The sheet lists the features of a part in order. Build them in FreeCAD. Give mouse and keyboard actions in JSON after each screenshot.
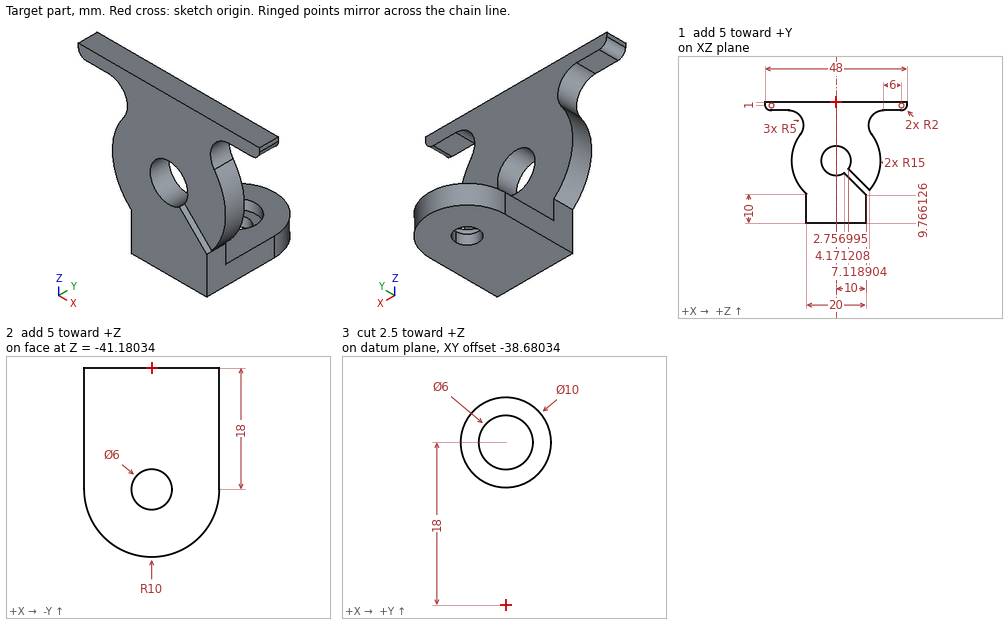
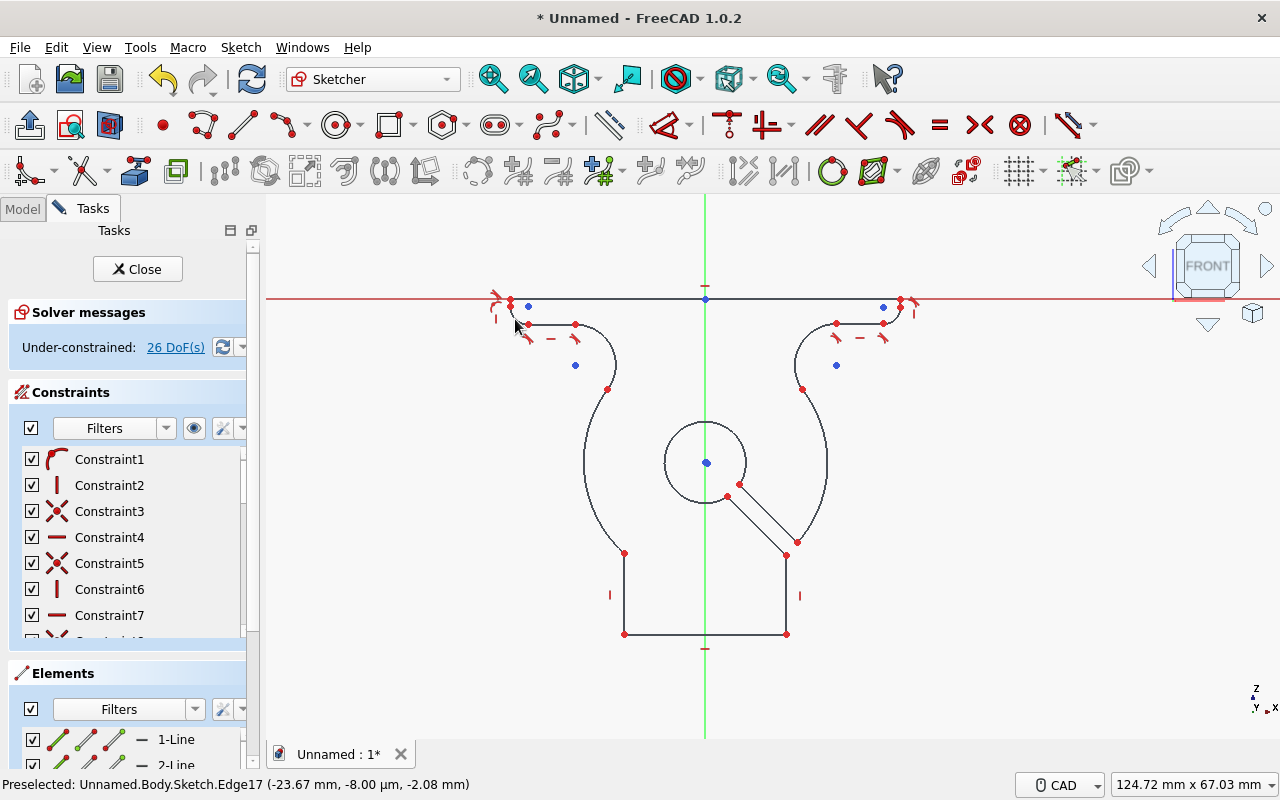
{"action": "left_click", "coordinate": [811, 333]}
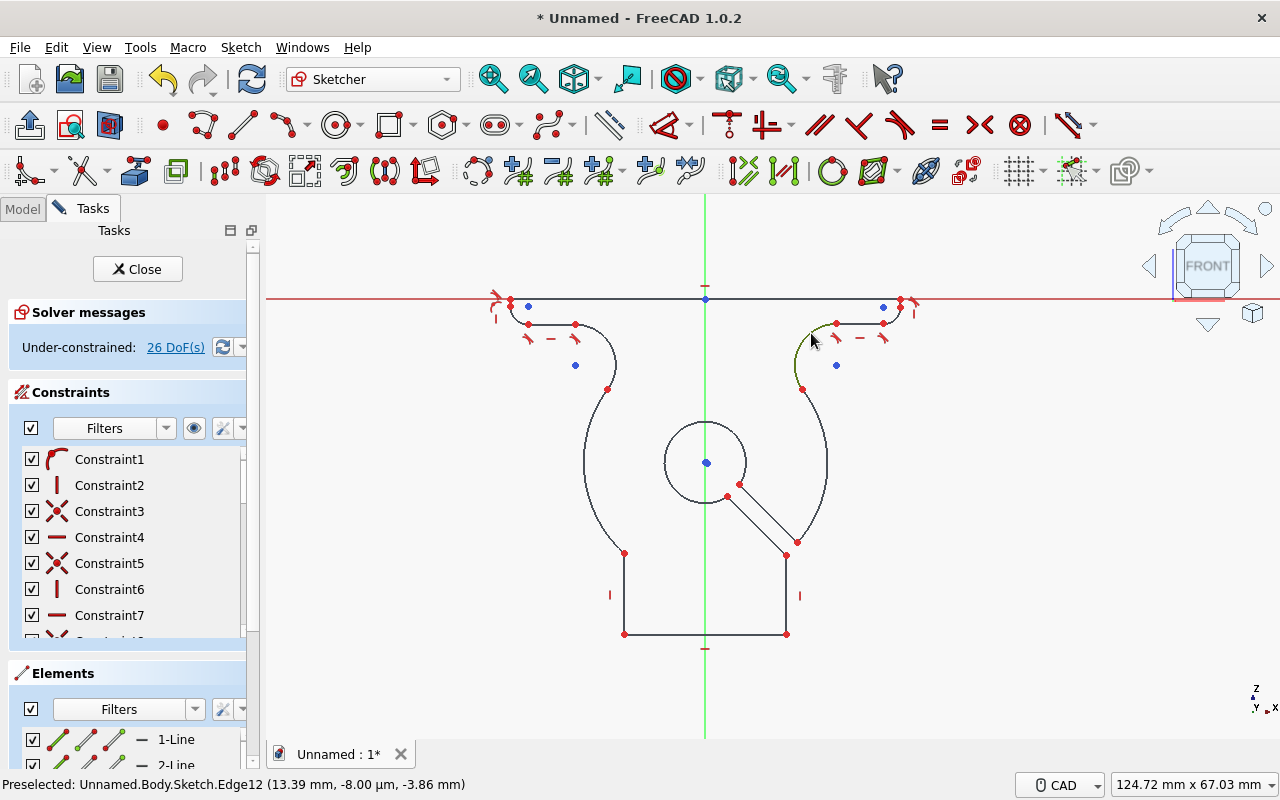
{"action": "left_click", "coordinate": [822, 500]}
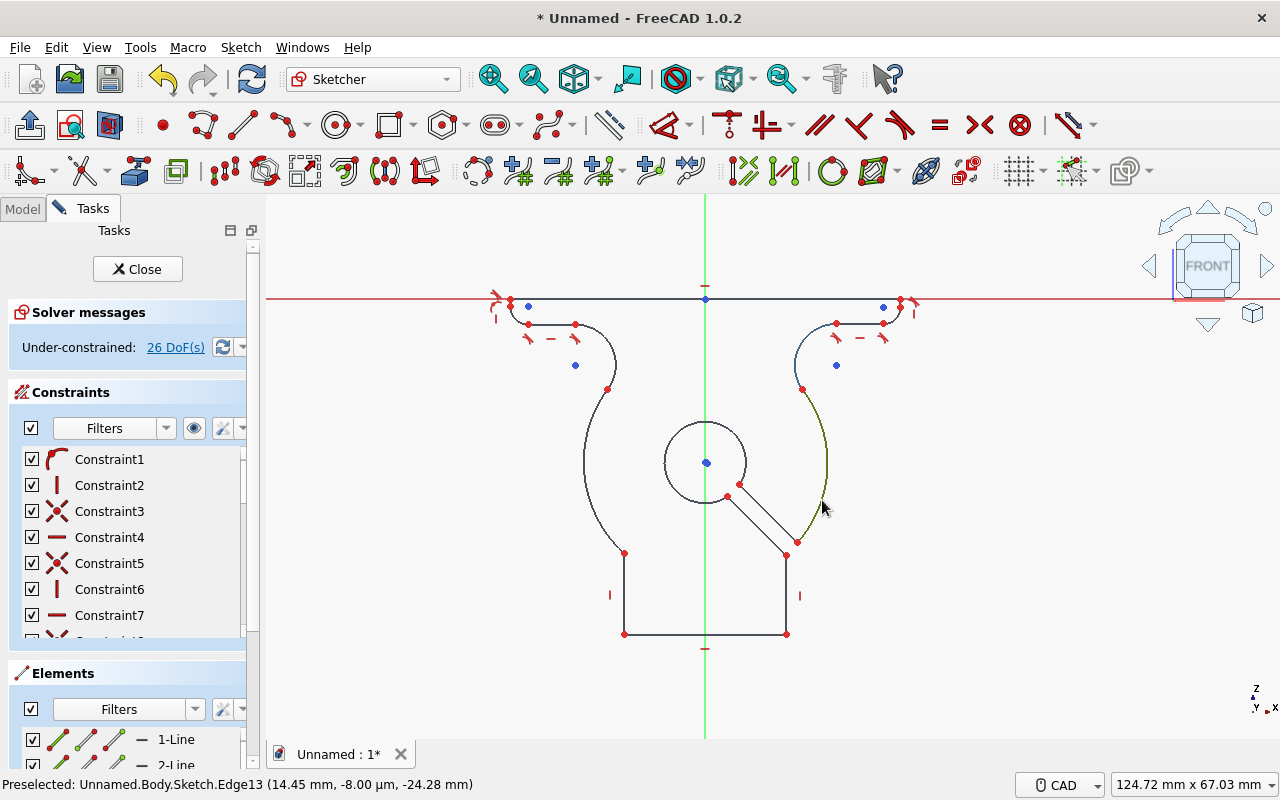
{"action": "left_click", "coordinate": [900, 126]}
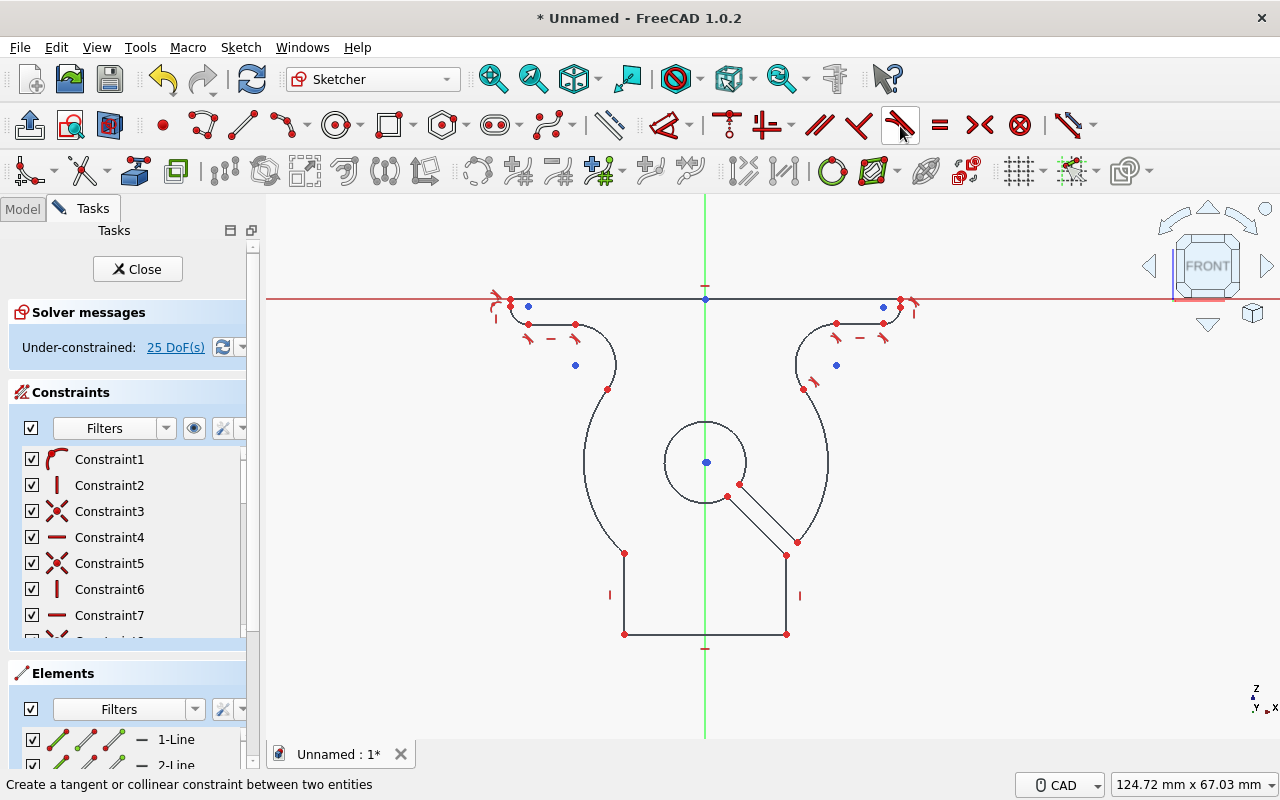
{"action": "left_click", "coordinate": [586, 439]}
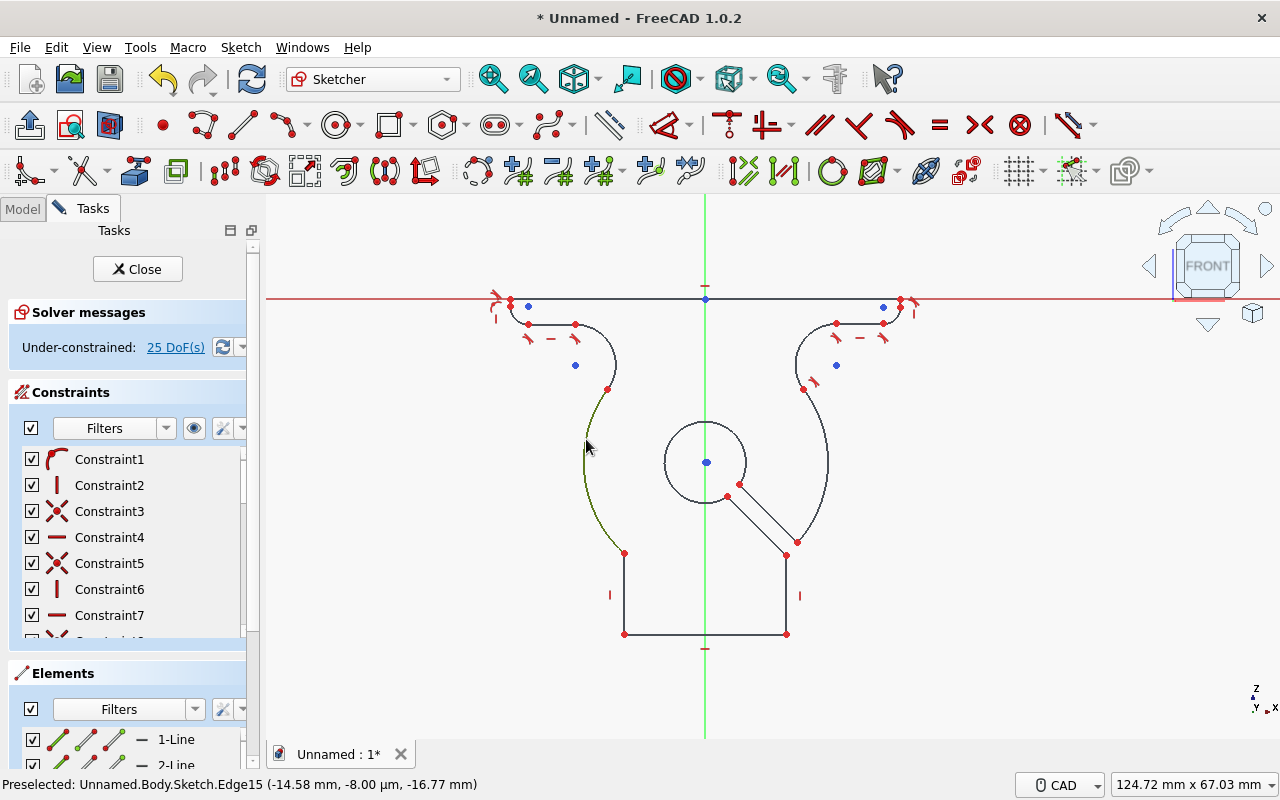
{"action": "left_click", "coordinate": [616, 365]}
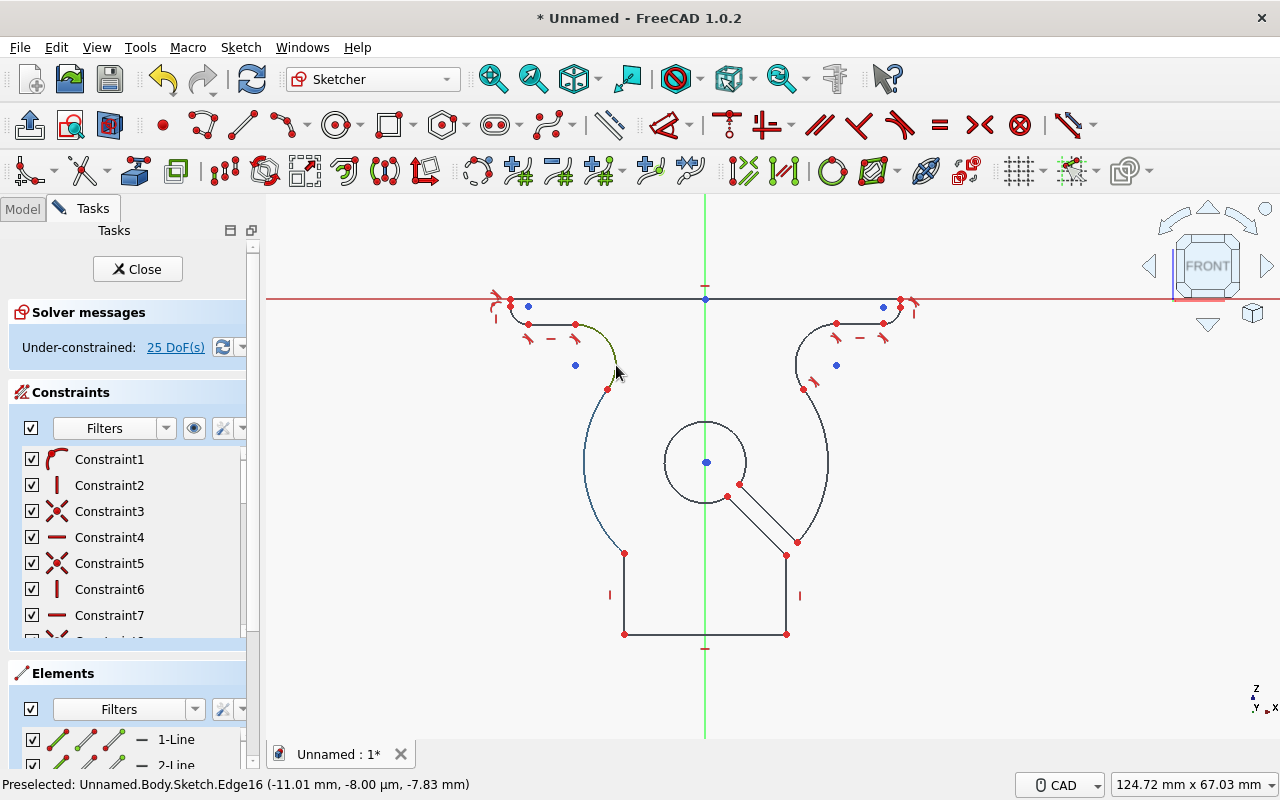
{"action": "key", "text": "t"}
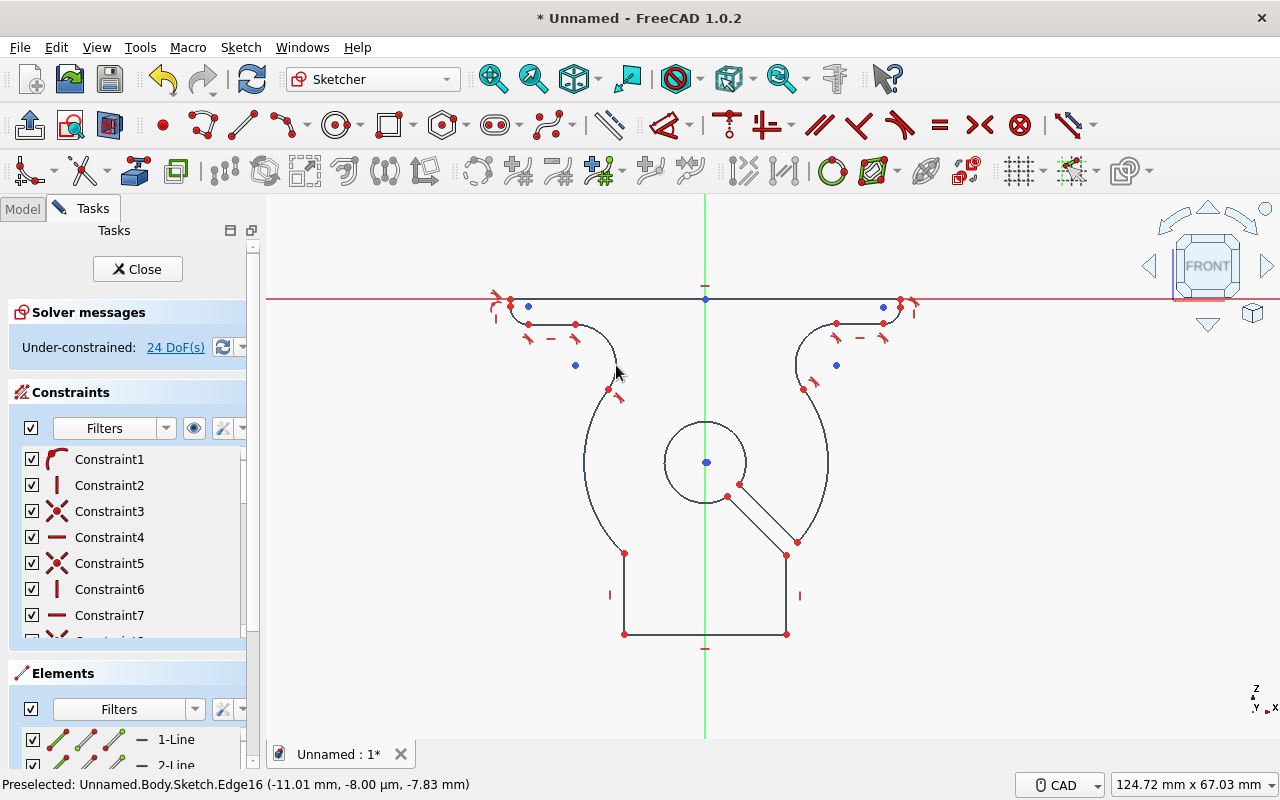
{"action": "left_click", "coordinate": [822, 500]}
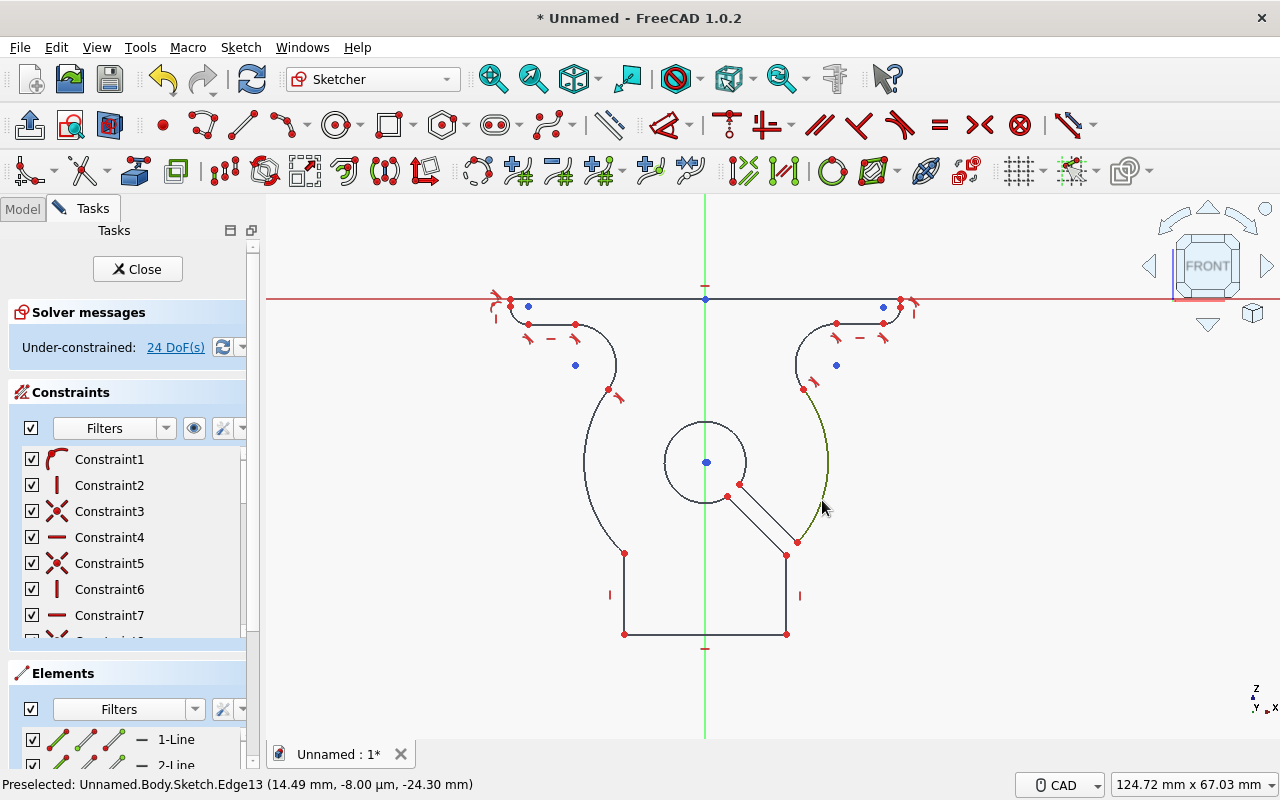
{"action": "left_click", "coordinate": [721, 425]}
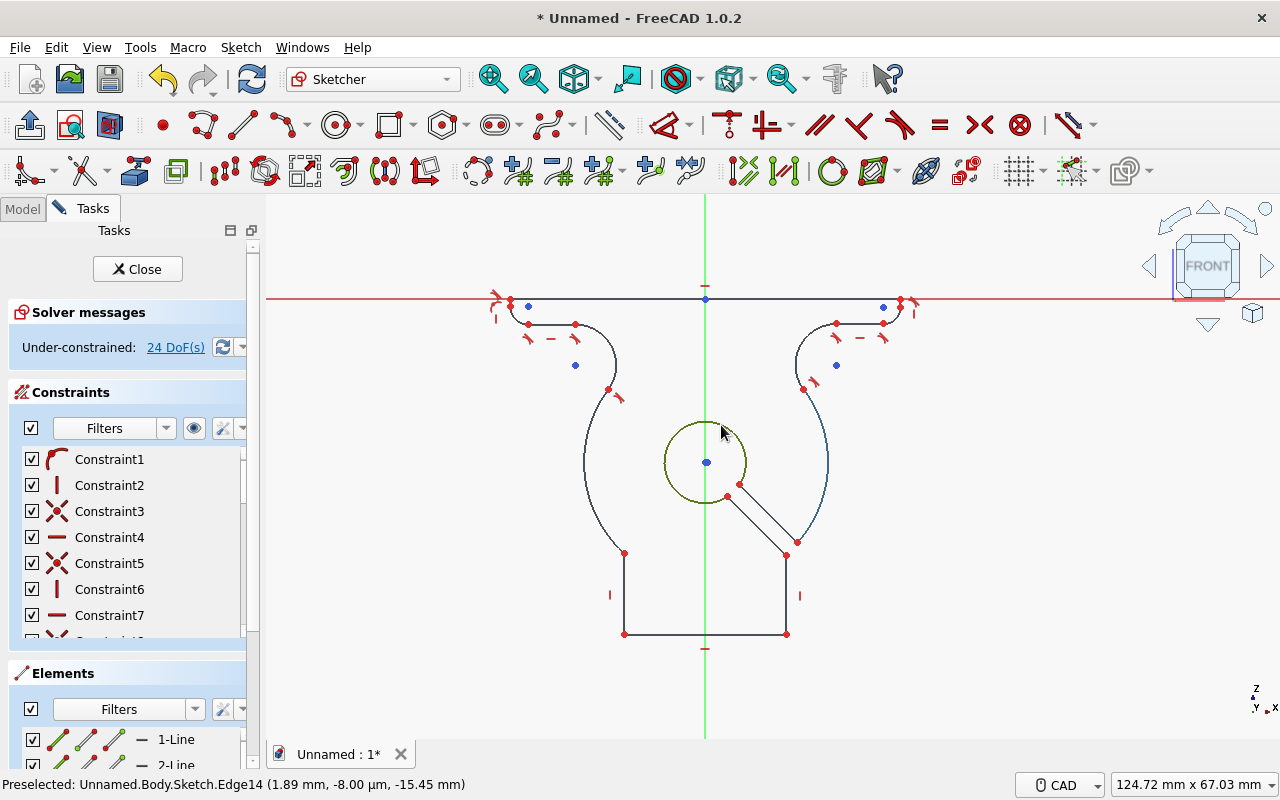
{"action": "key", "text": "c"}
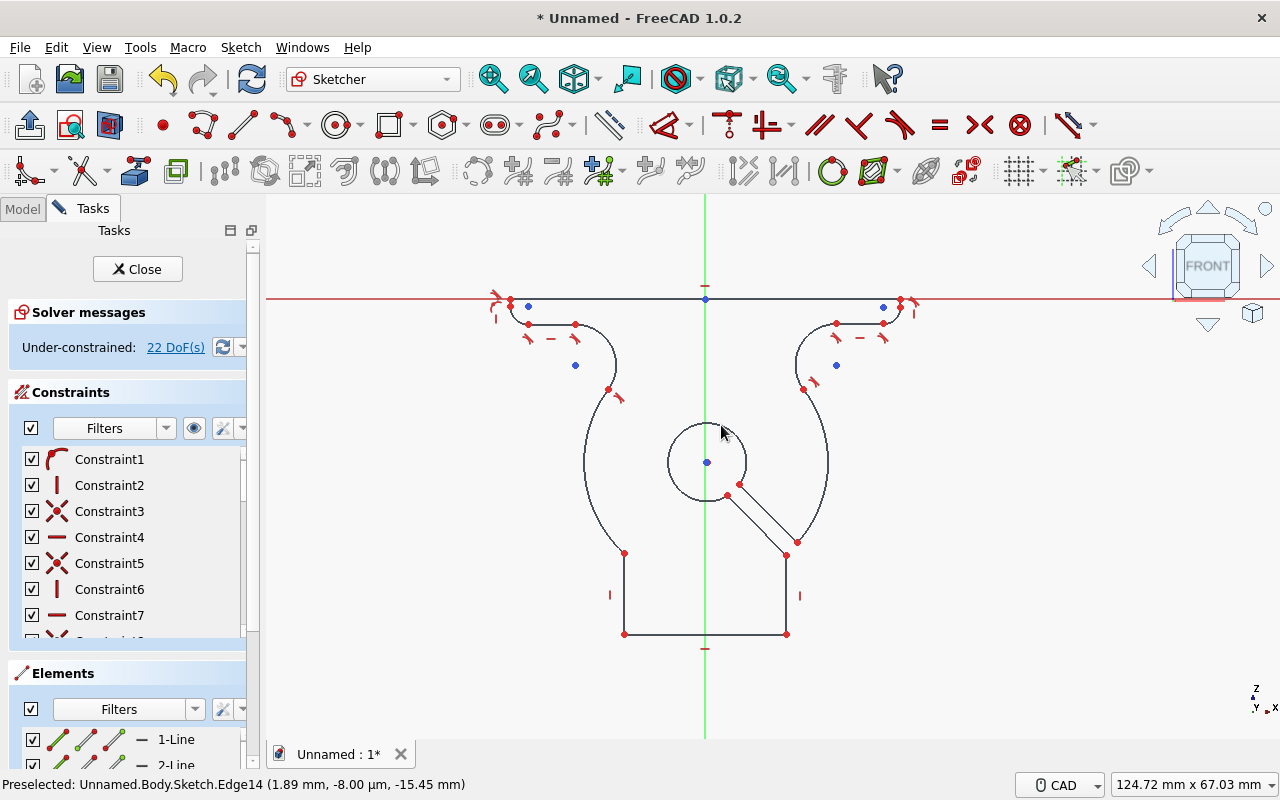
{"action": "left_click", "coordinate": [822, 500]}